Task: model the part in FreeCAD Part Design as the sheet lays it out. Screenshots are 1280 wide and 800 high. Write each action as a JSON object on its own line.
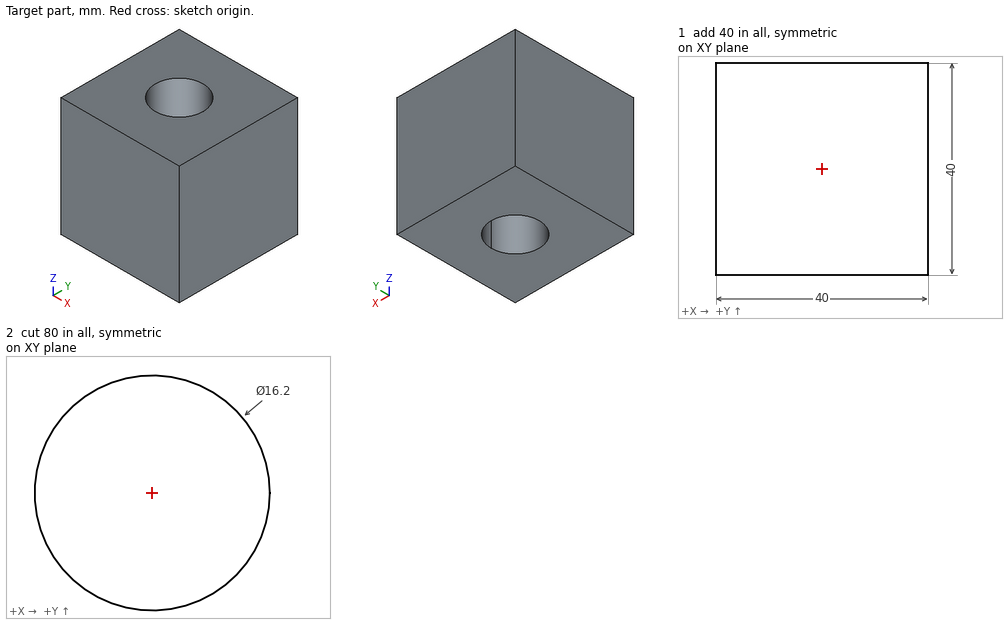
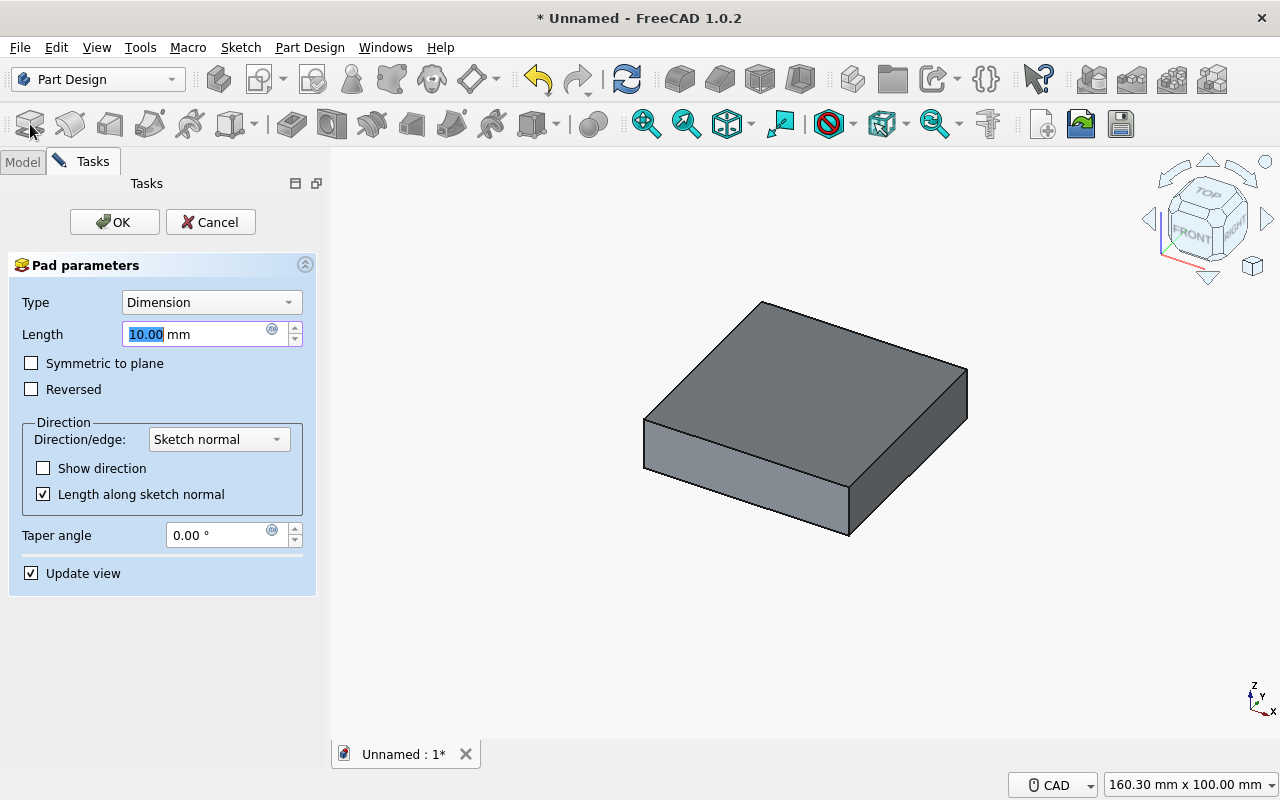
{"action": "type", "text": "40"}
{"action": "key", "text": "Tab"}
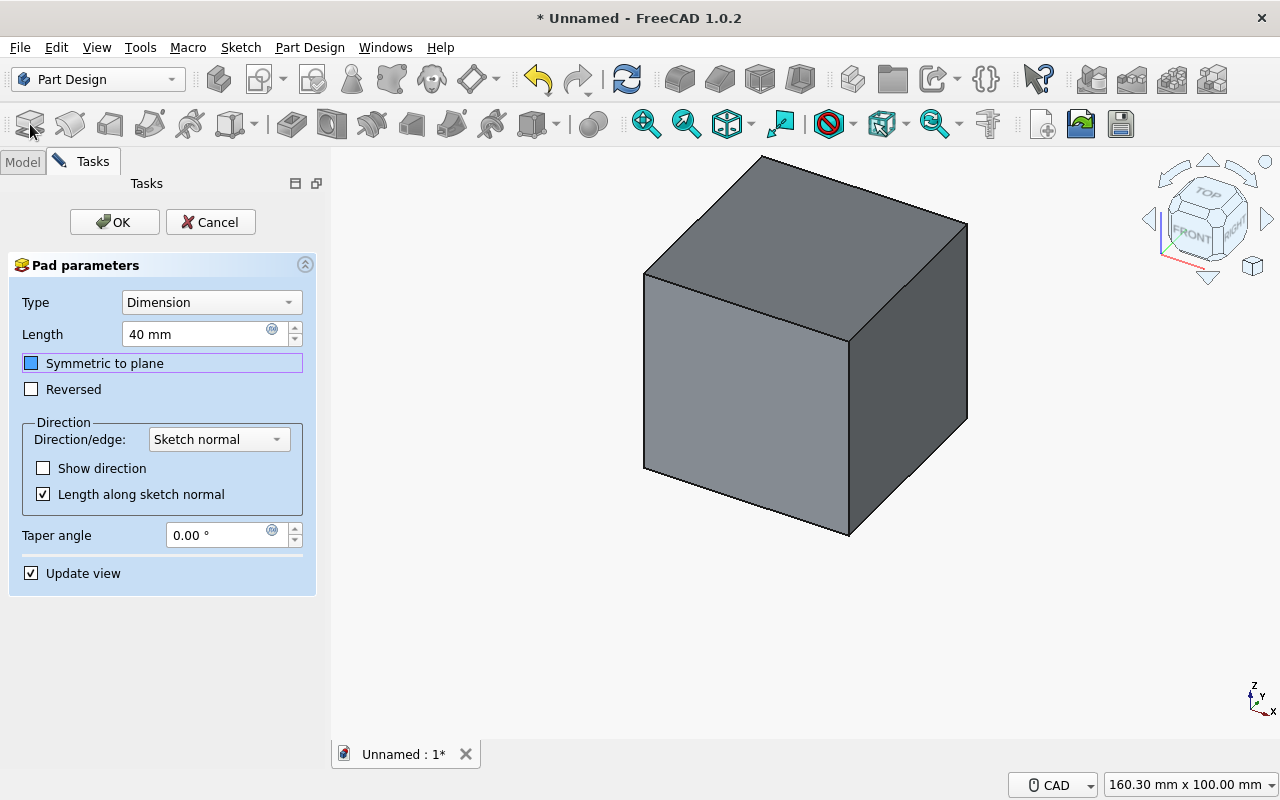
{"action": "left_click", "coordinate": [30, 363]}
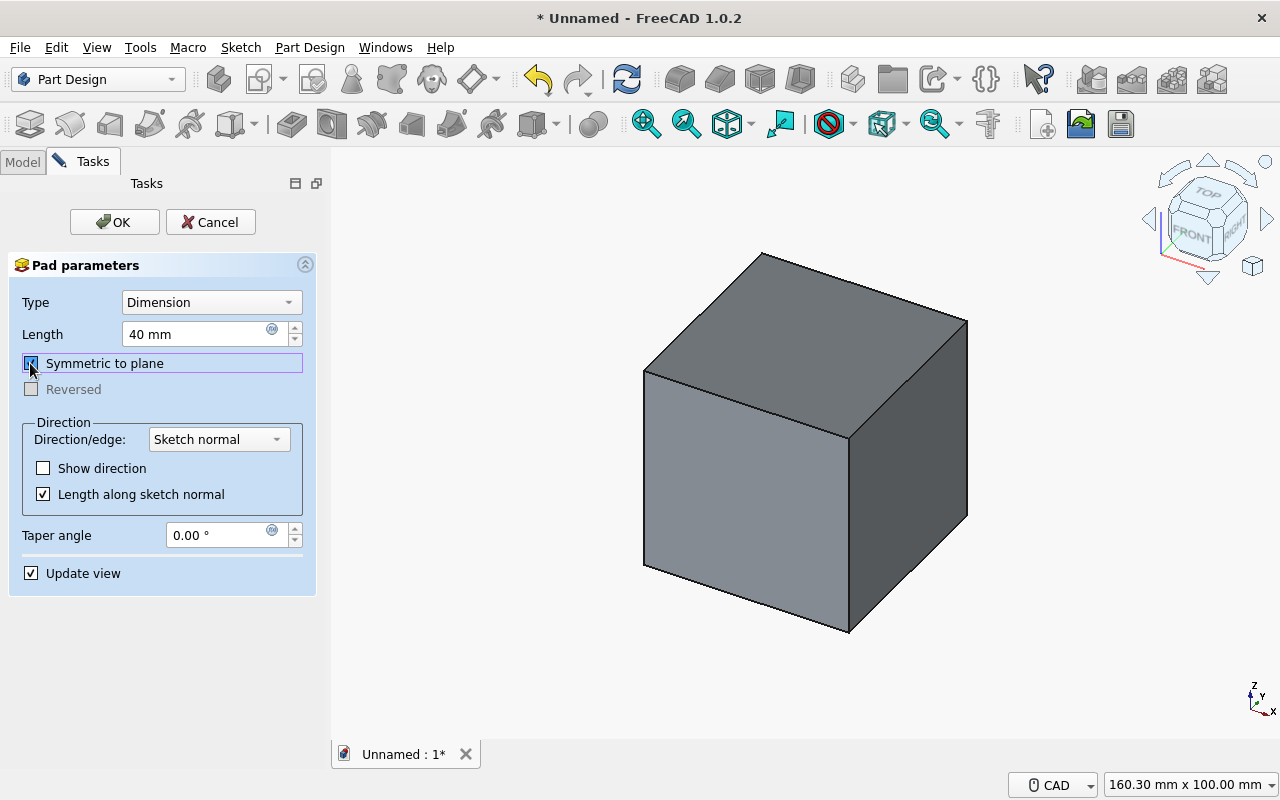
{"action": "left_click", "coordinate": [115, 222]}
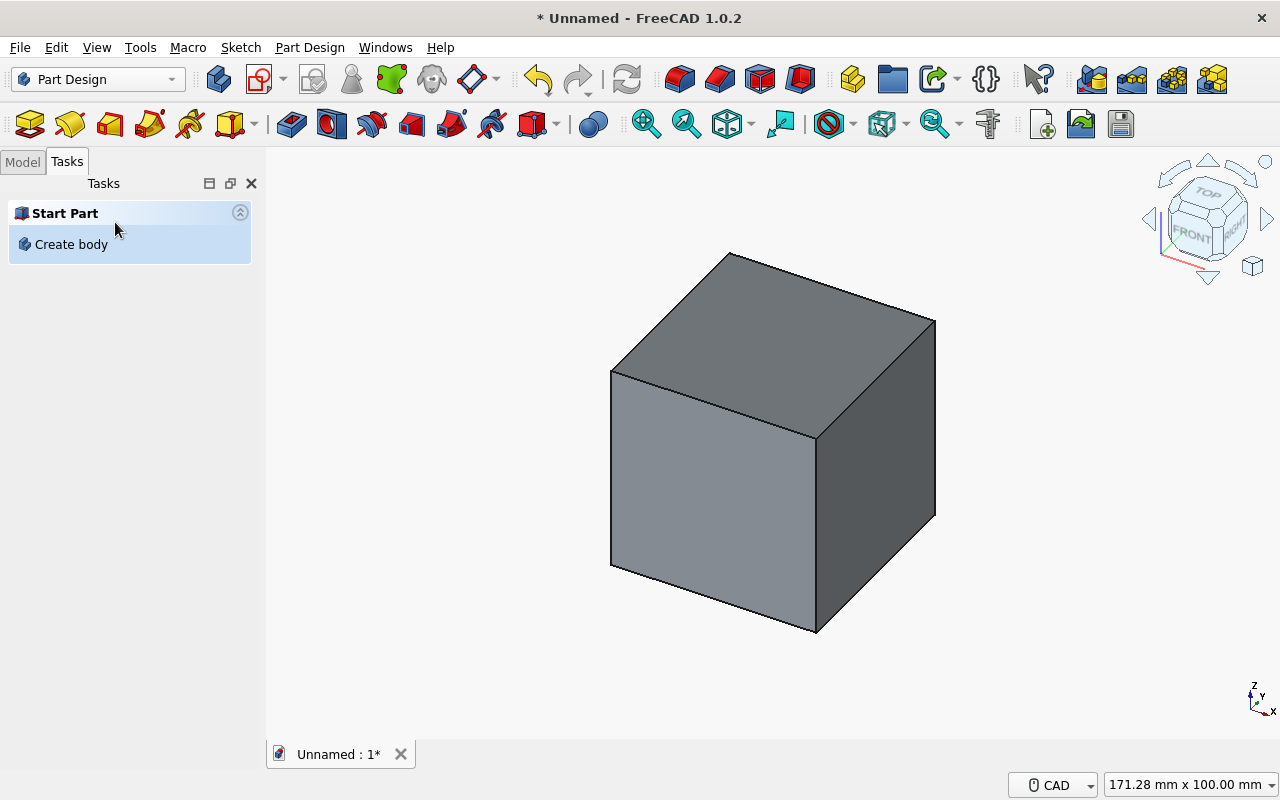
{"action": "left_click", "coordinate": [260, 80]}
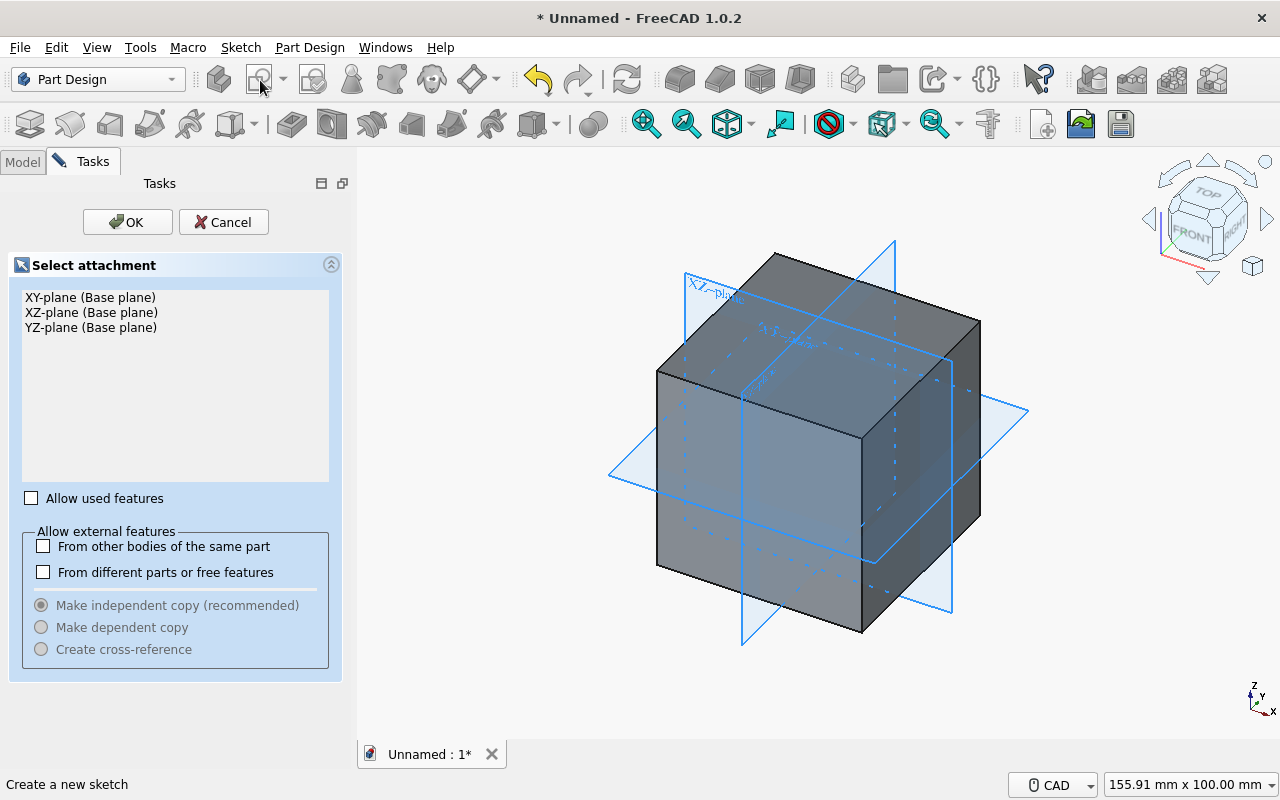
{"action": "left_click", "coordinate": [82, 298]}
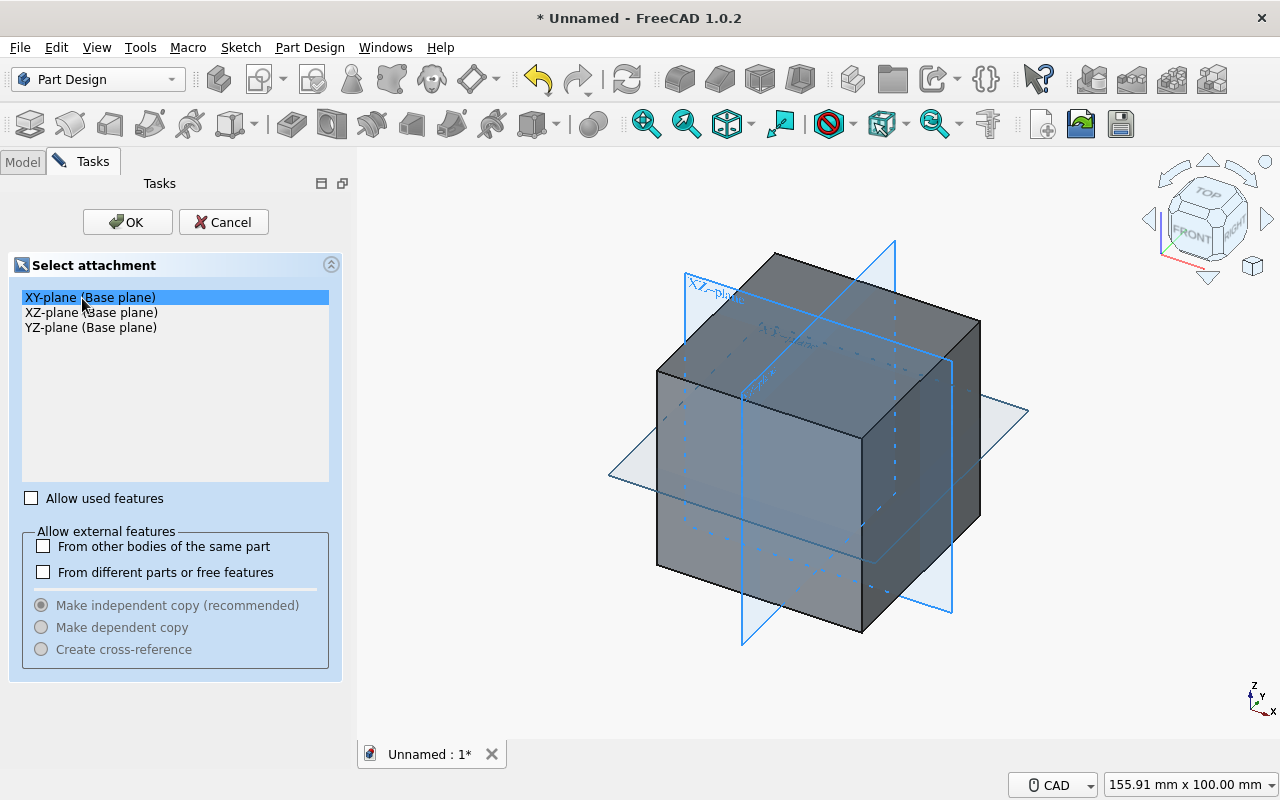
{"action": "left_click", "coordinate": [128, 222]}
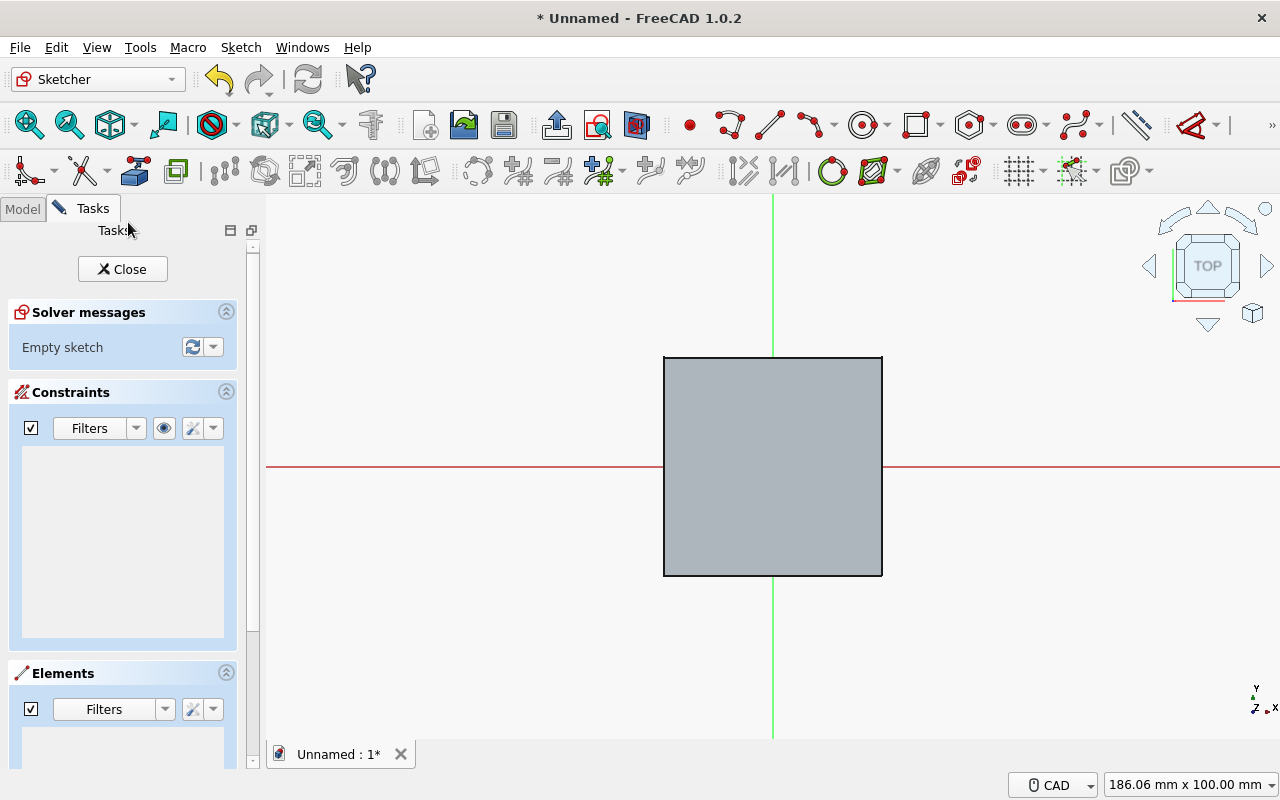
{"action": "key", "text": "q s"}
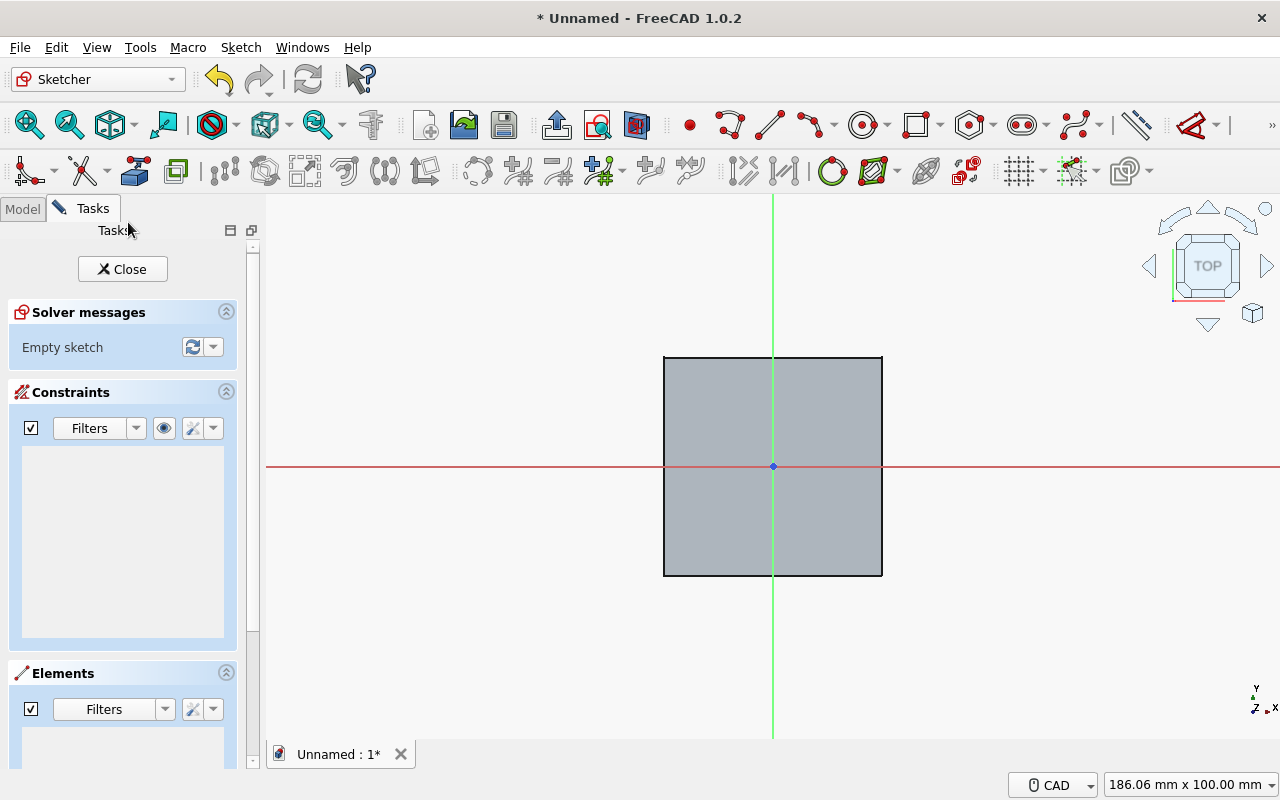
{"action": "scroll", "coordinate": [795, 466], "scroll_direction": "up", "scroll_amount": 7}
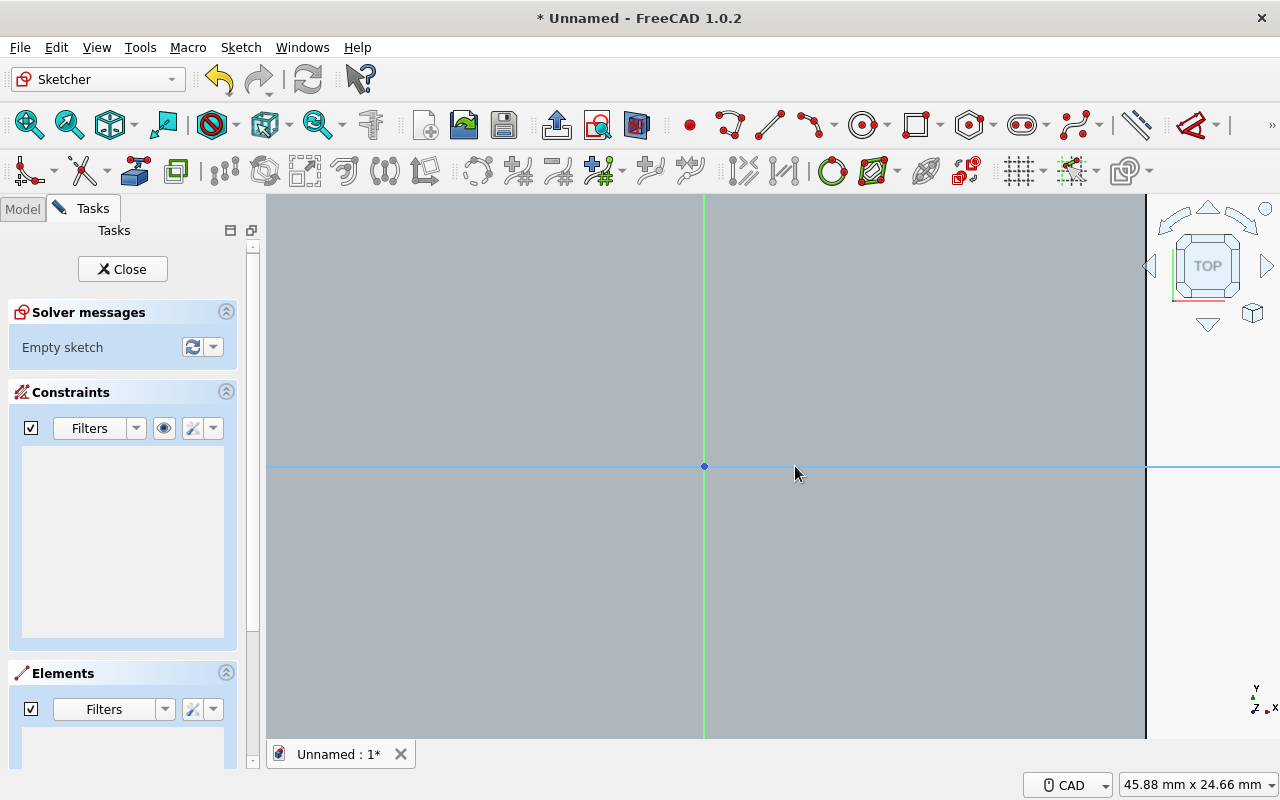
{"action": "key", "text": "g c"}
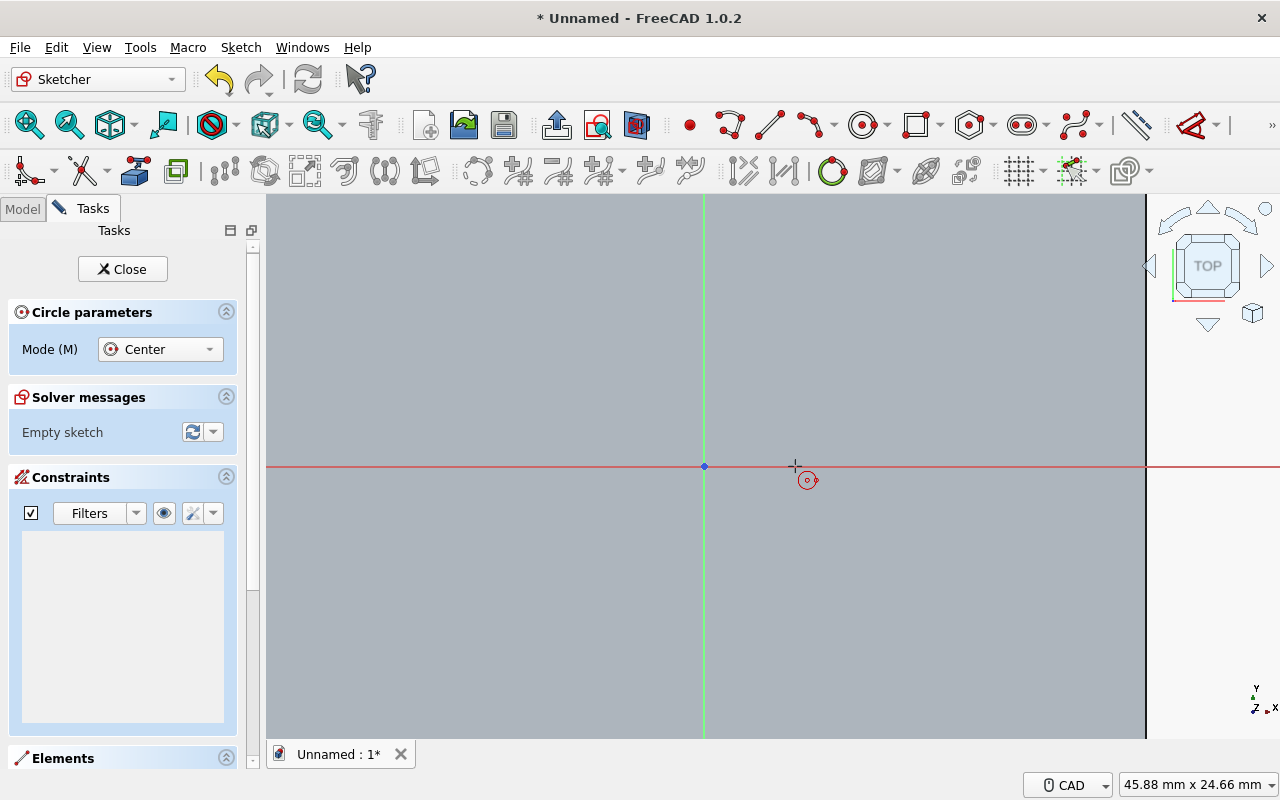
{"action": "left_click", "coordinate": [704, 466]}
{"action": "mouse_move", "coordinate": [831, 340]}